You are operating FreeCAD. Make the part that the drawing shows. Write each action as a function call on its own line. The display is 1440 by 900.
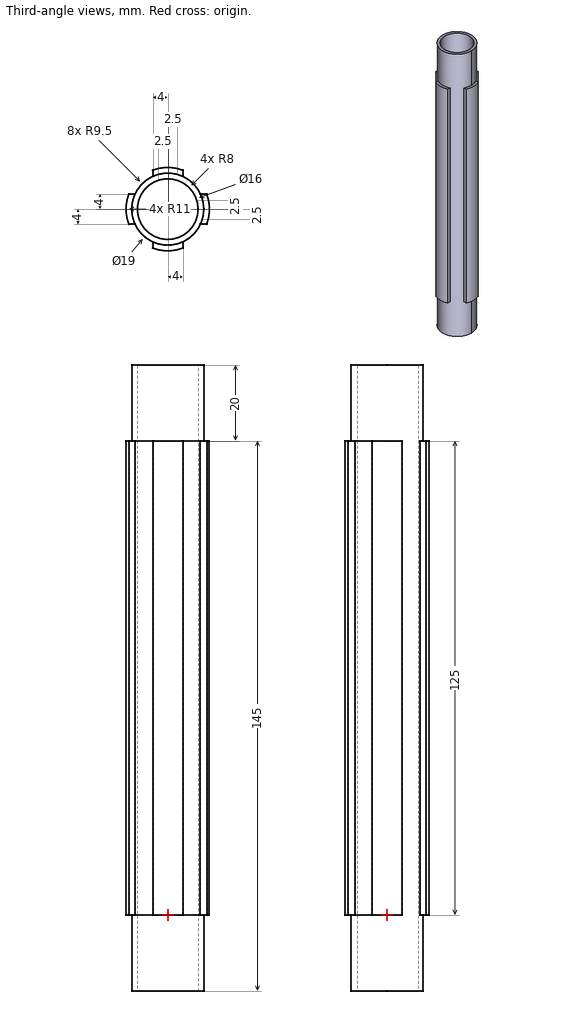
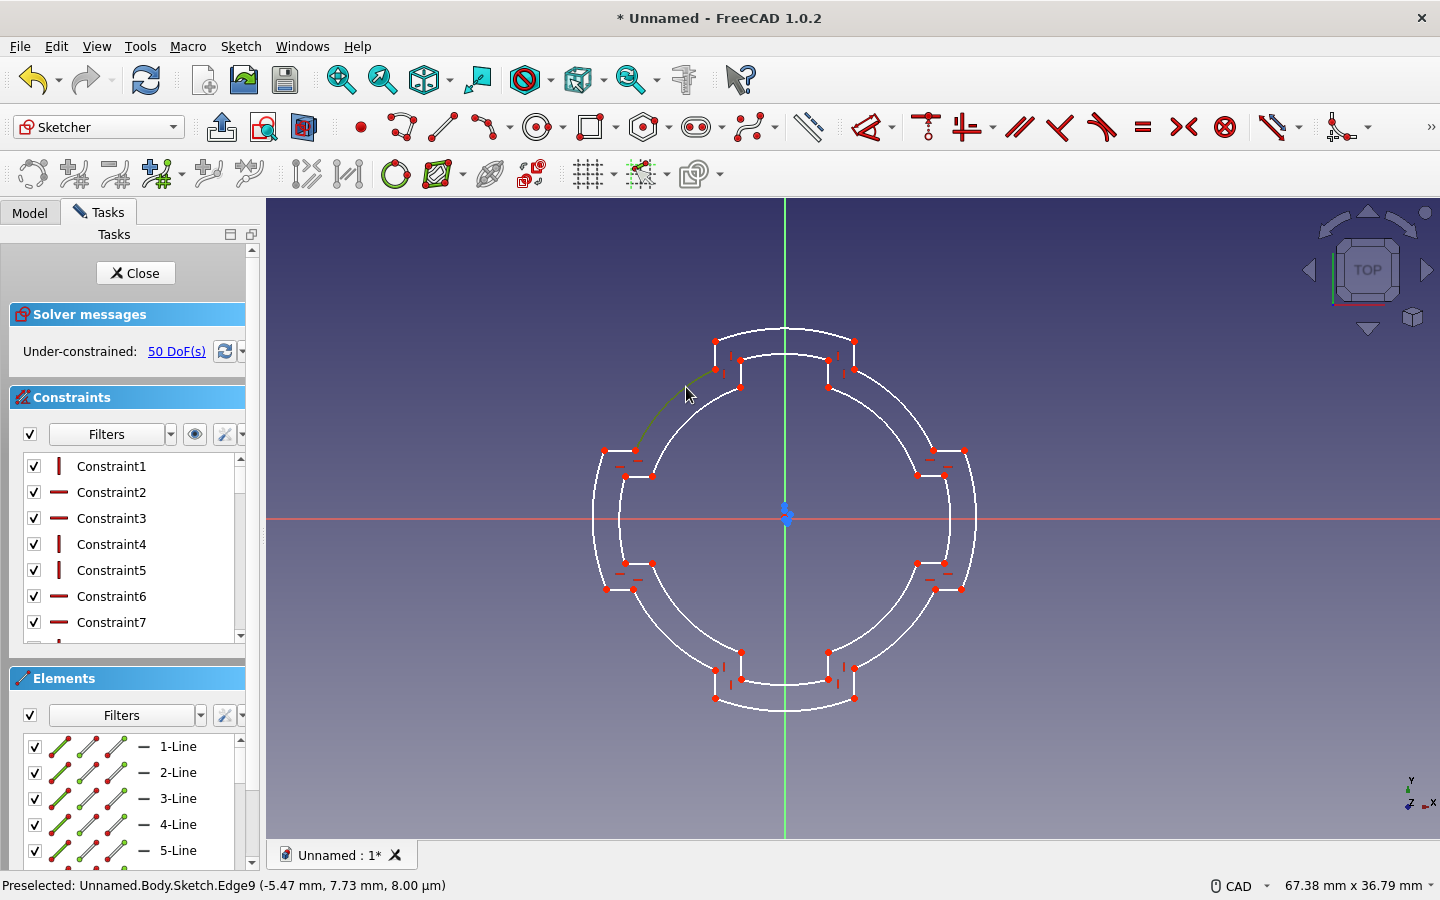
click(802, 355)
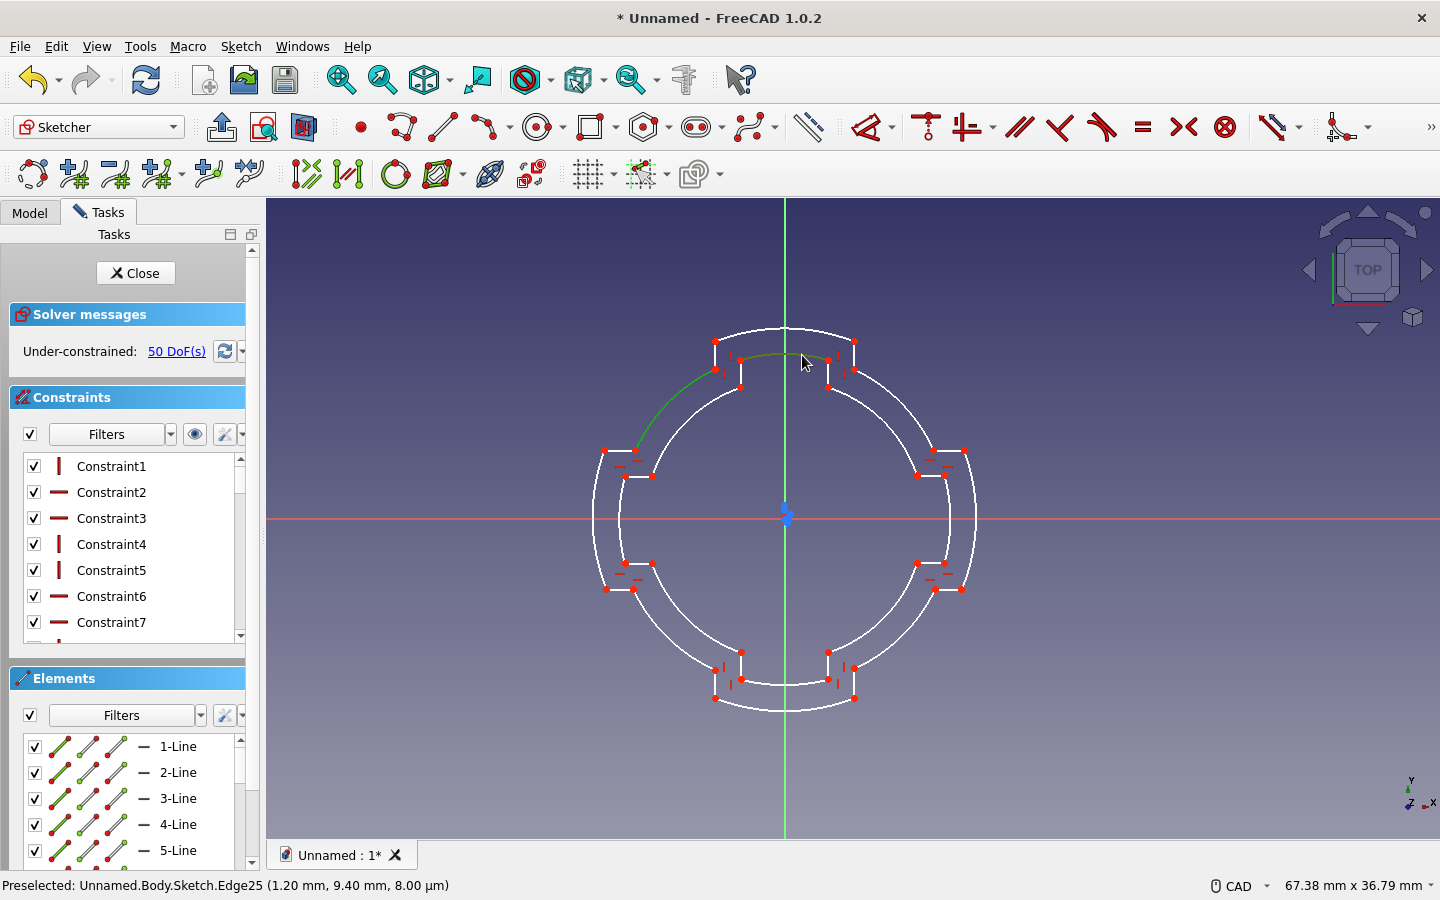
click(926, 128)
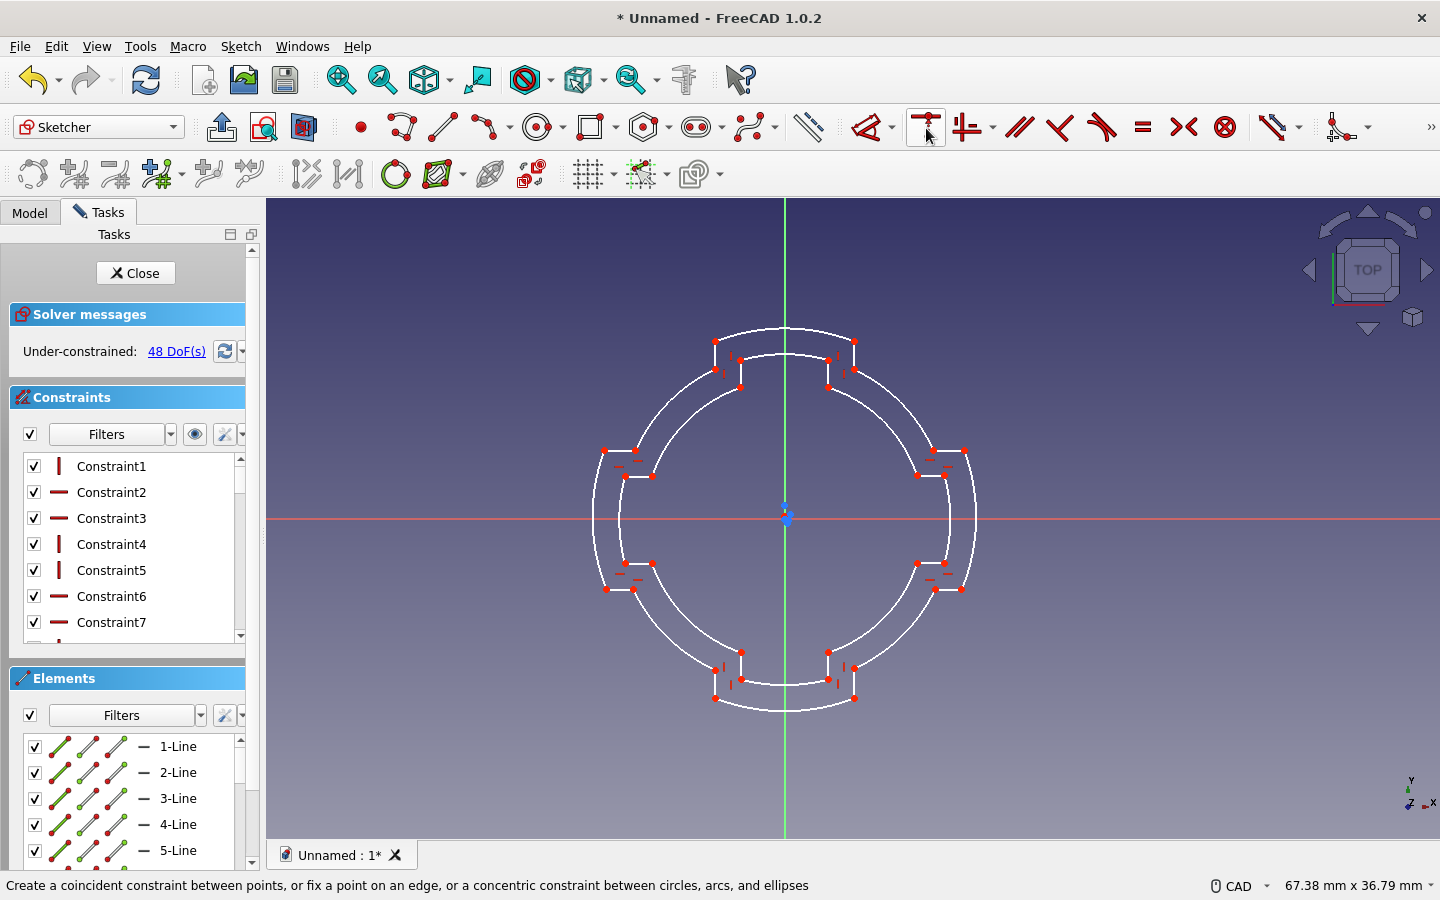
click(686, 387)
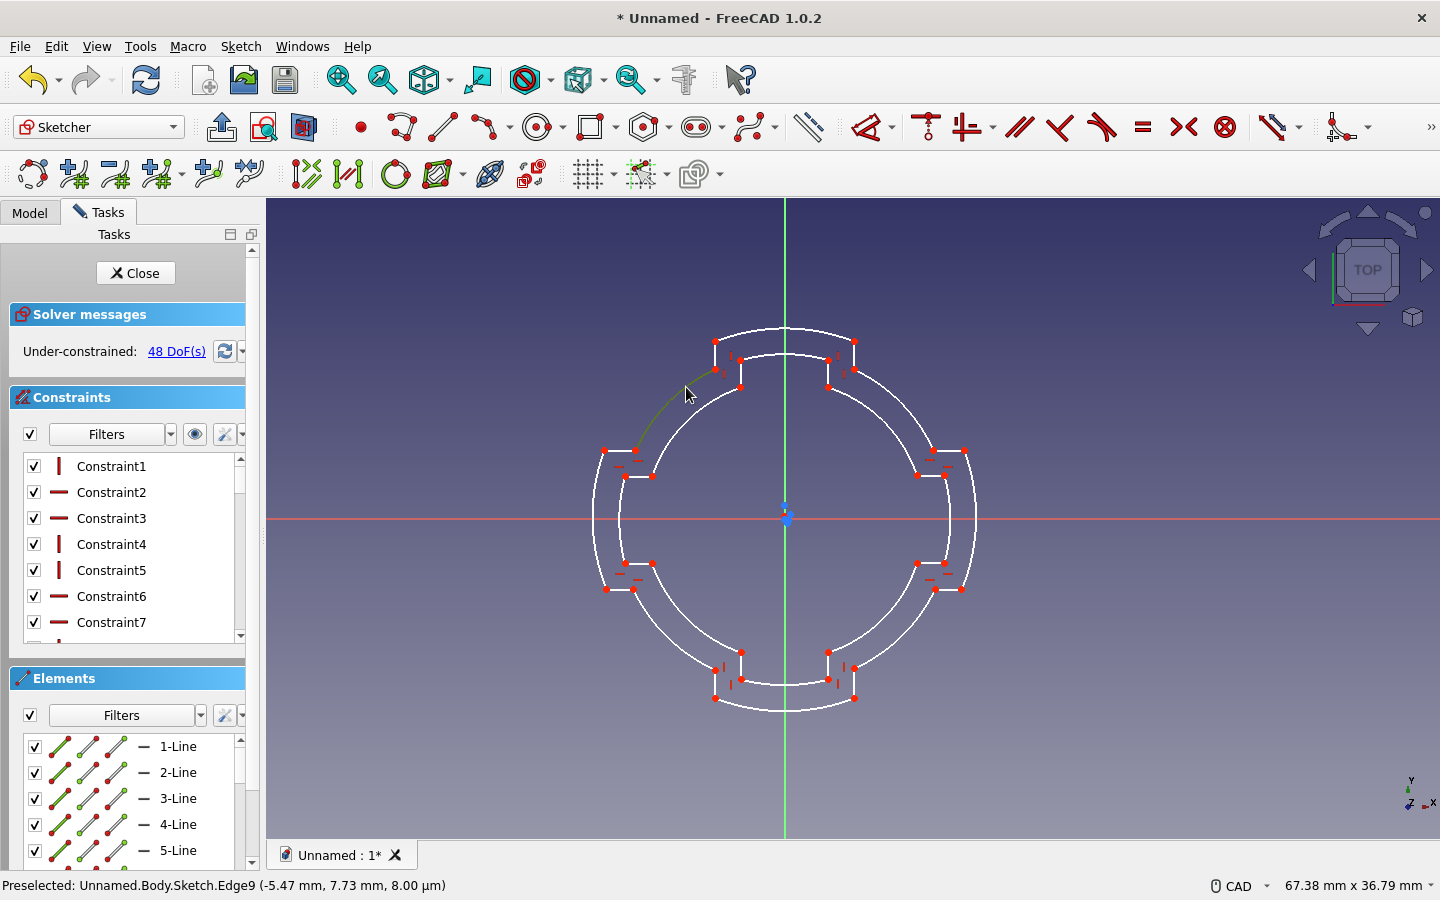
click(900, 441)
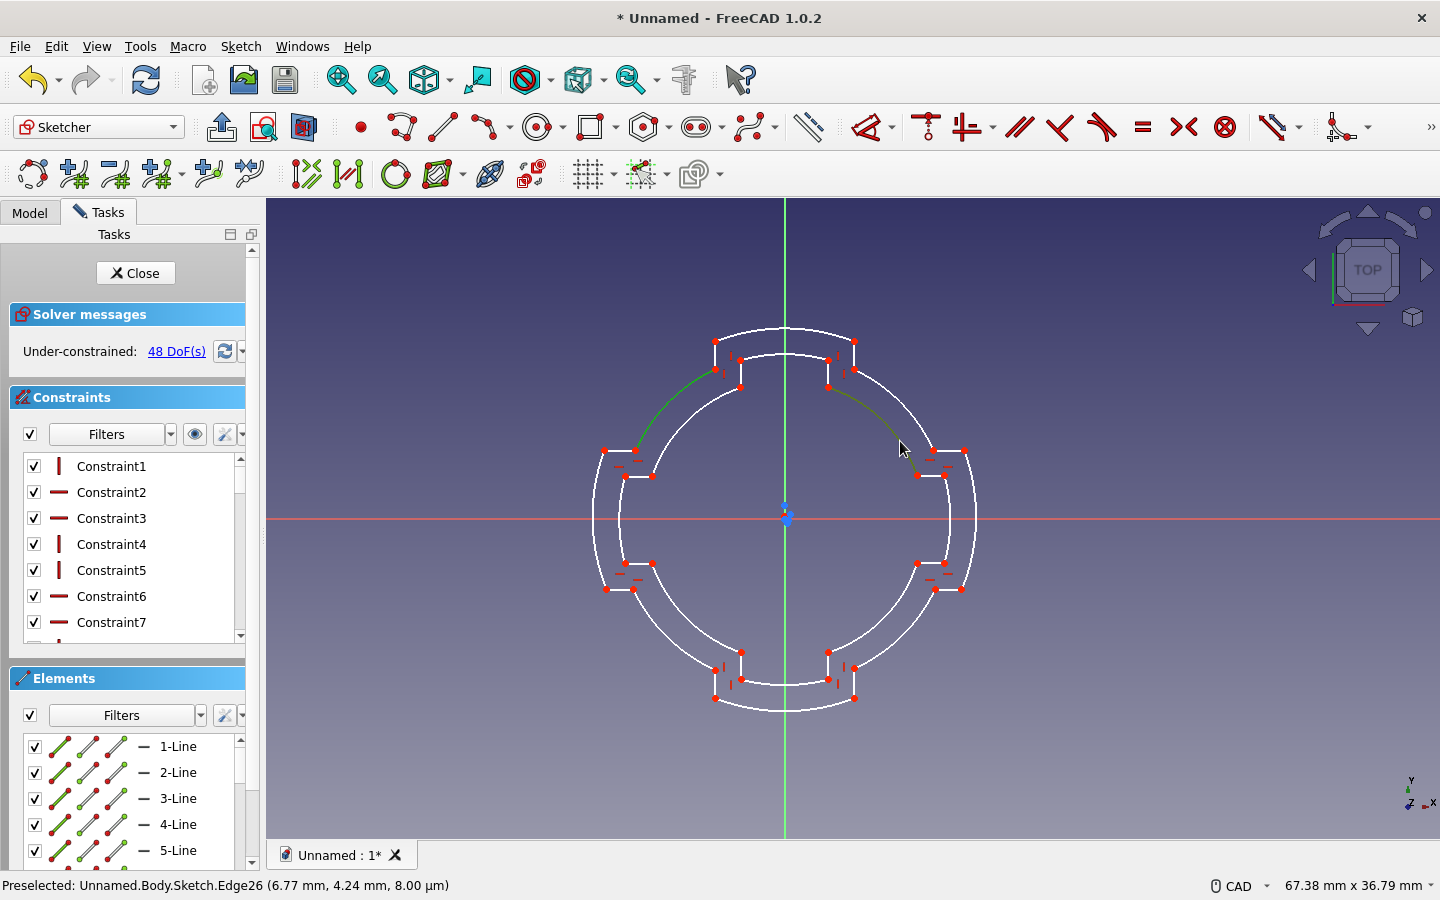
click(926, 128)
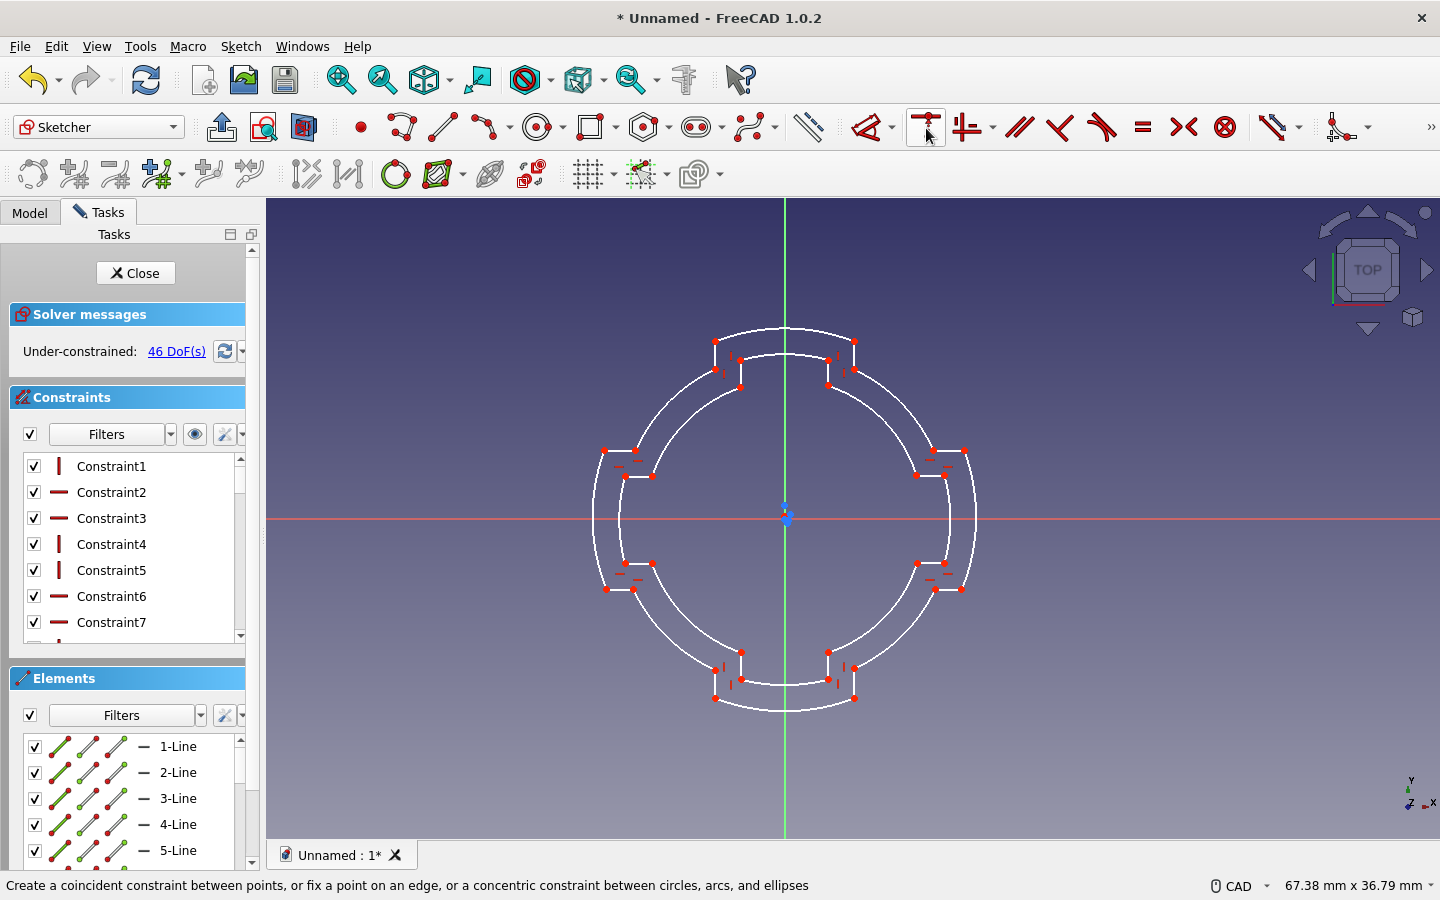
click(686, 387)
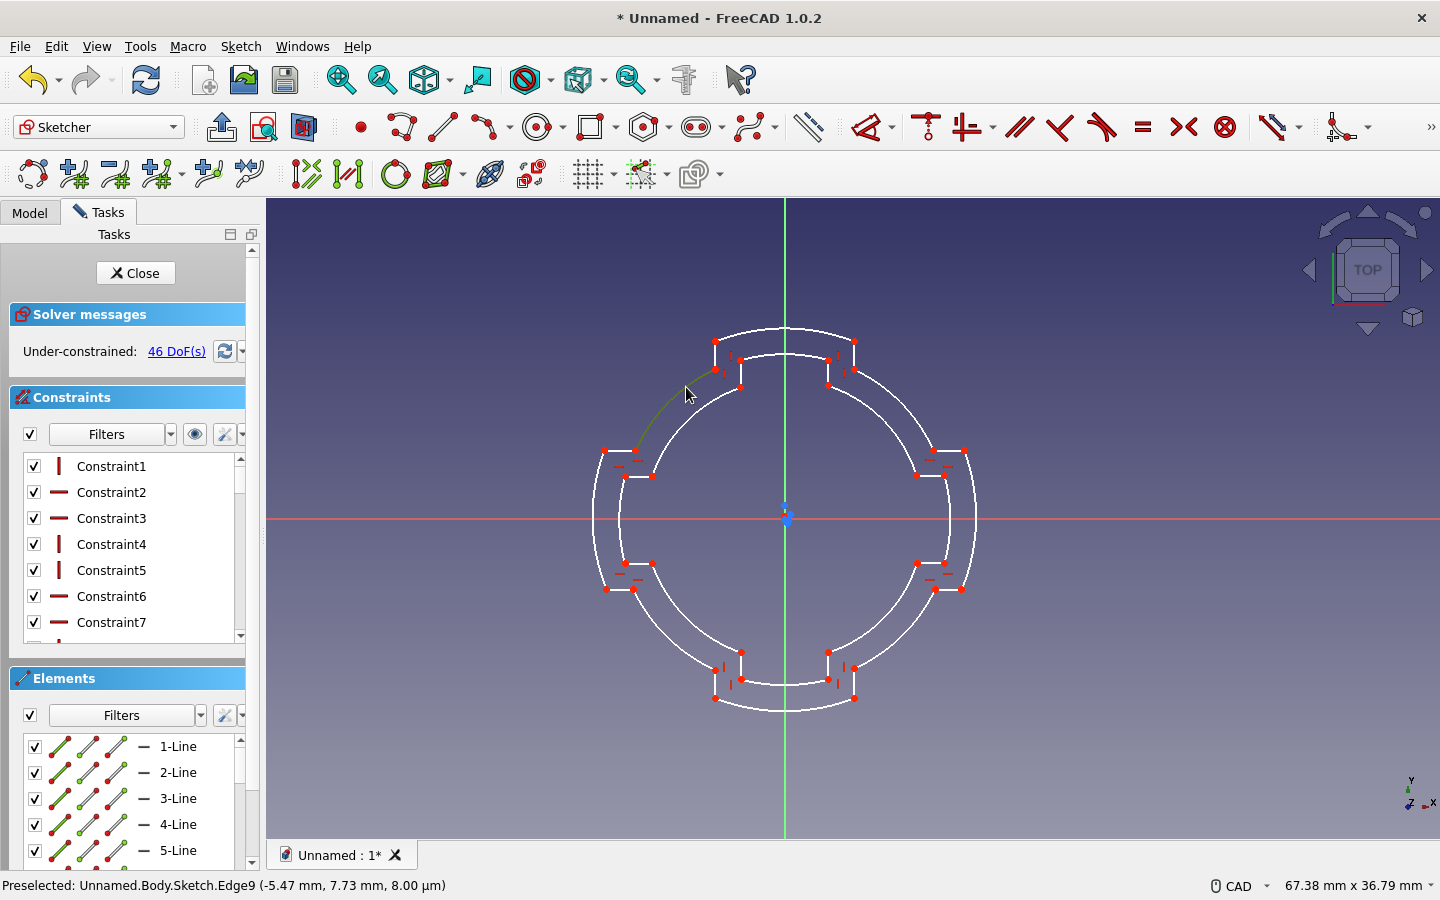
click(949, 537)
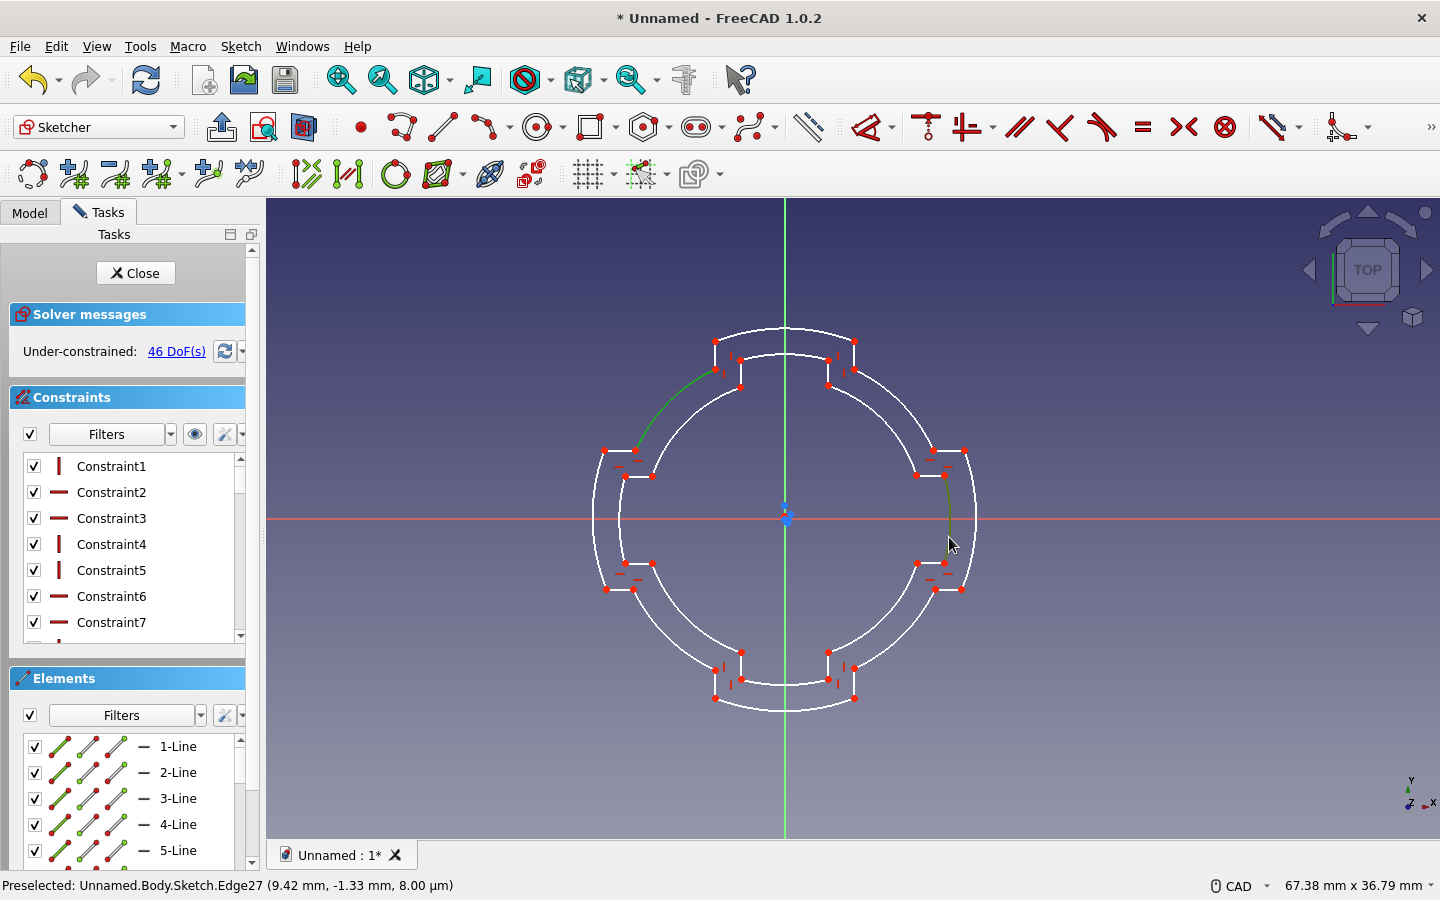
click(926, 128)